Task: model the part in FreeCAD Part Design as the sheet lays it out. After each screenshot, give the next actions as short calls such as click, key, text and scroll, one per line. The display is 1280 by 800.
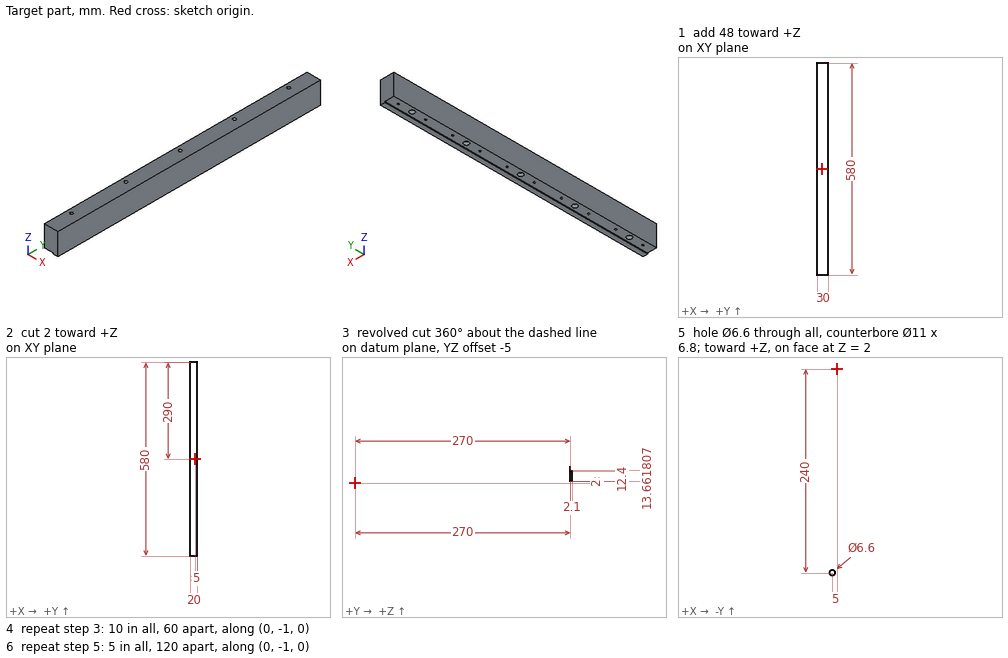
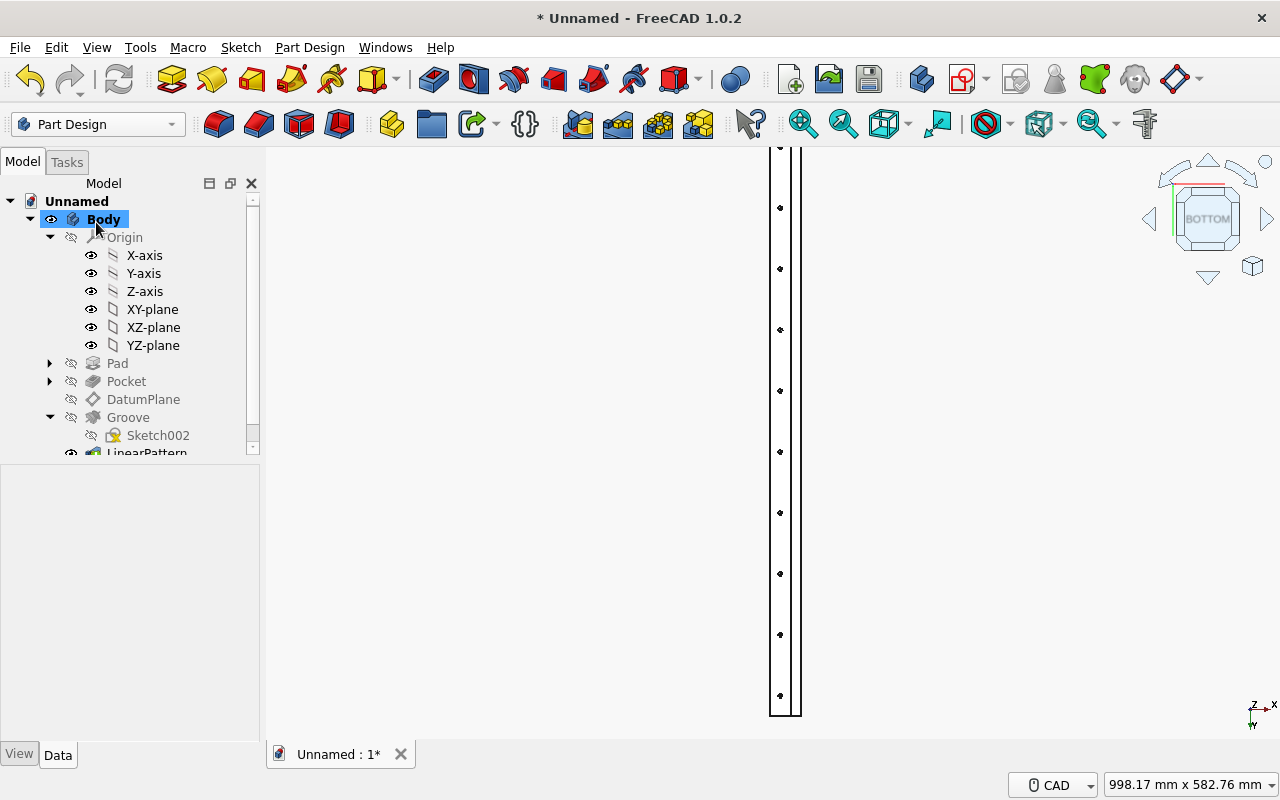
click(804, 124)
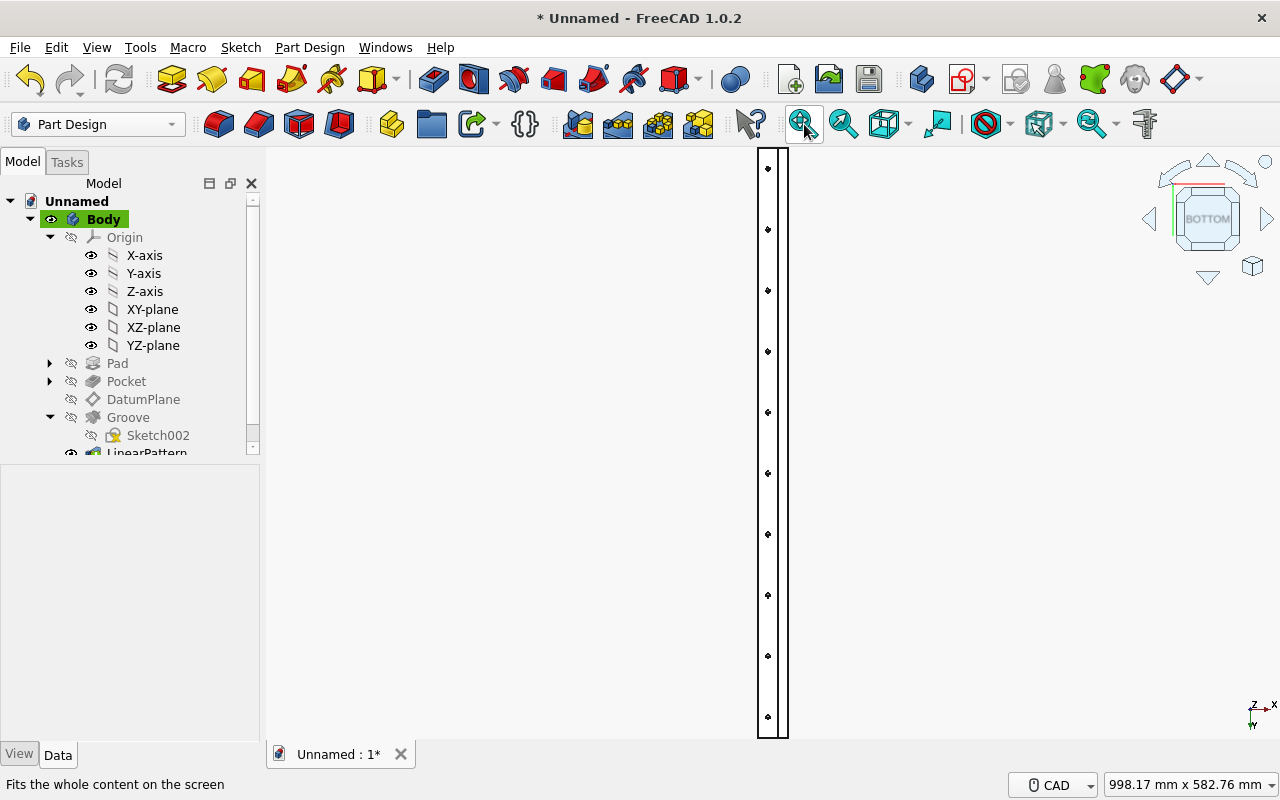
click(768, 695)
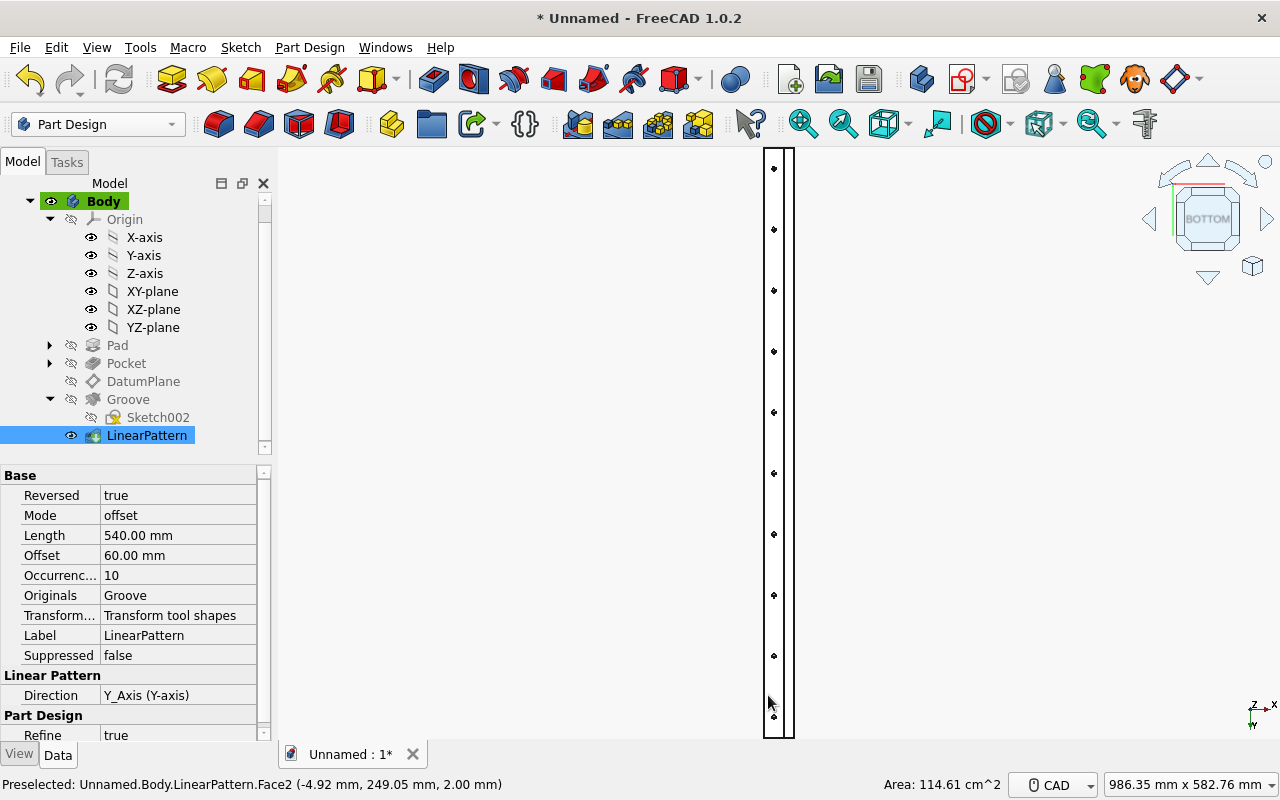
click(962, 80)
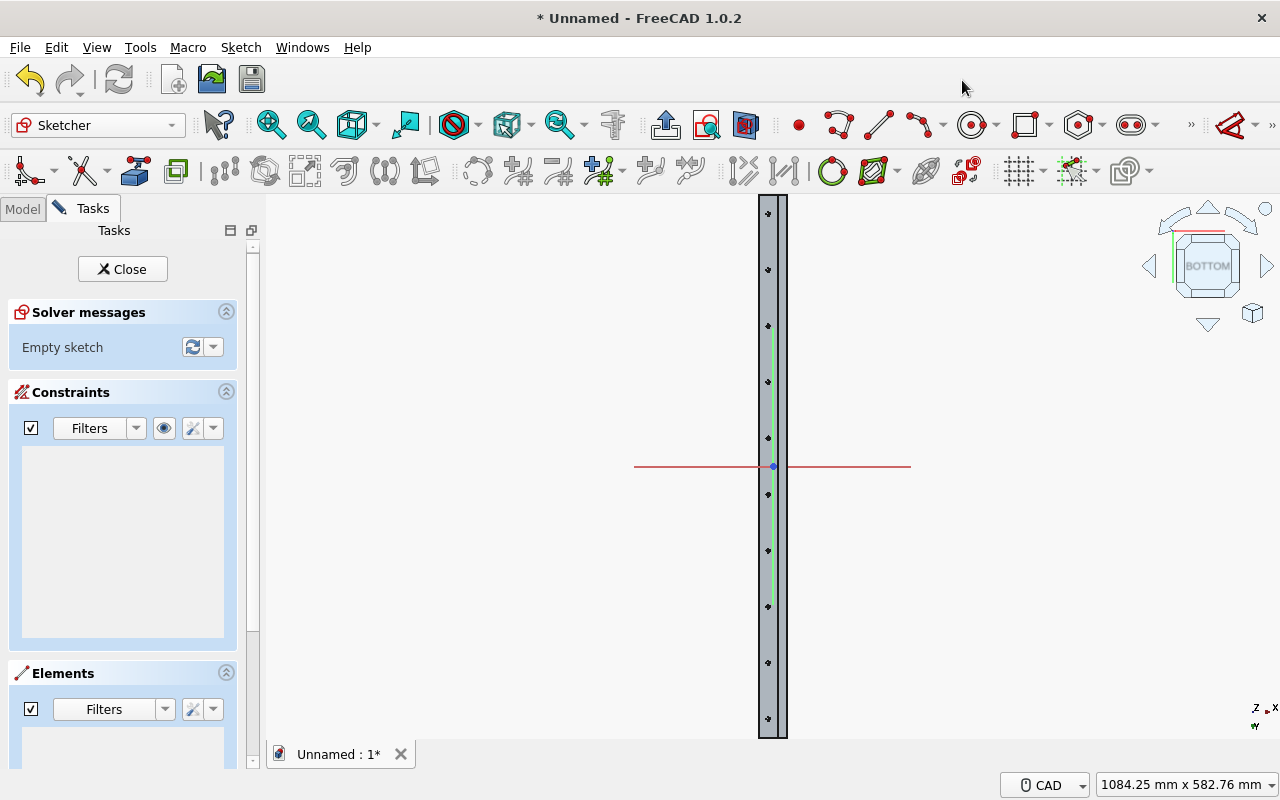
scroll(772, 703, up, 15)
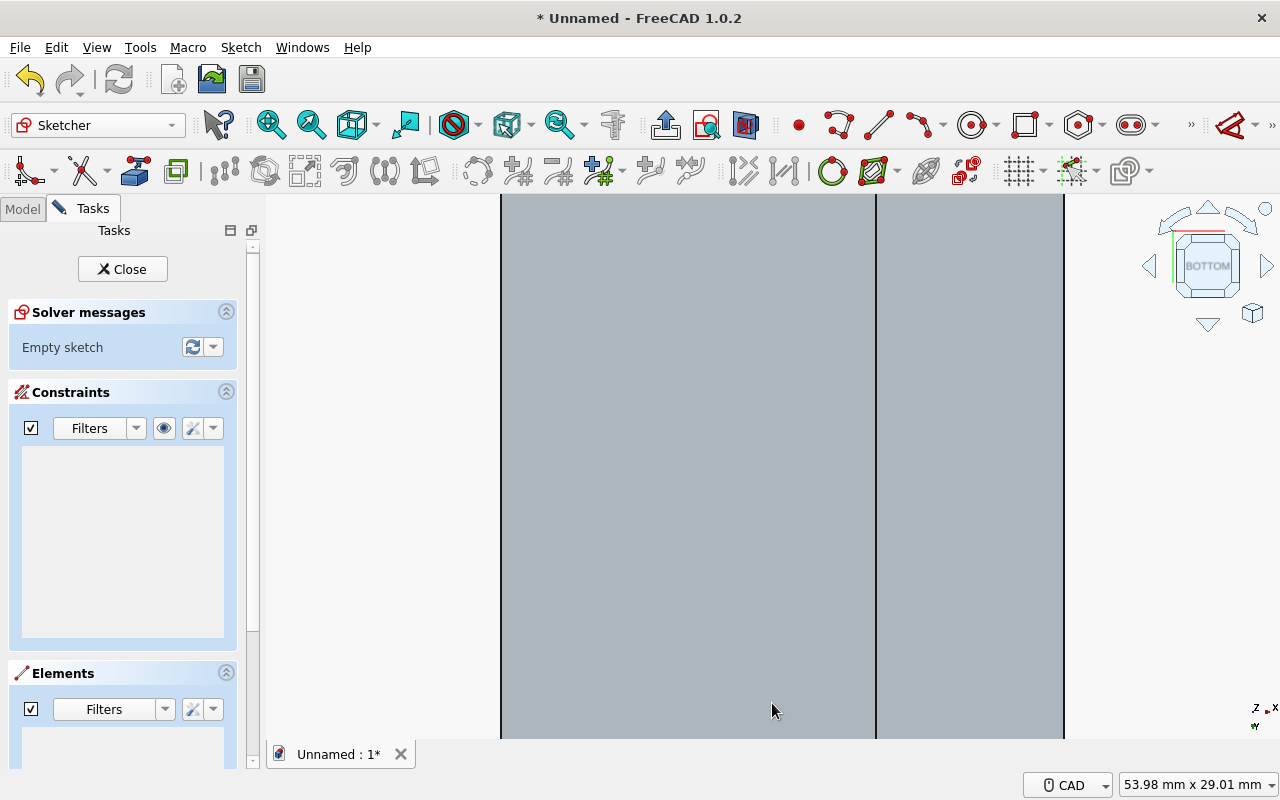
scroll(679, 430, up, 5)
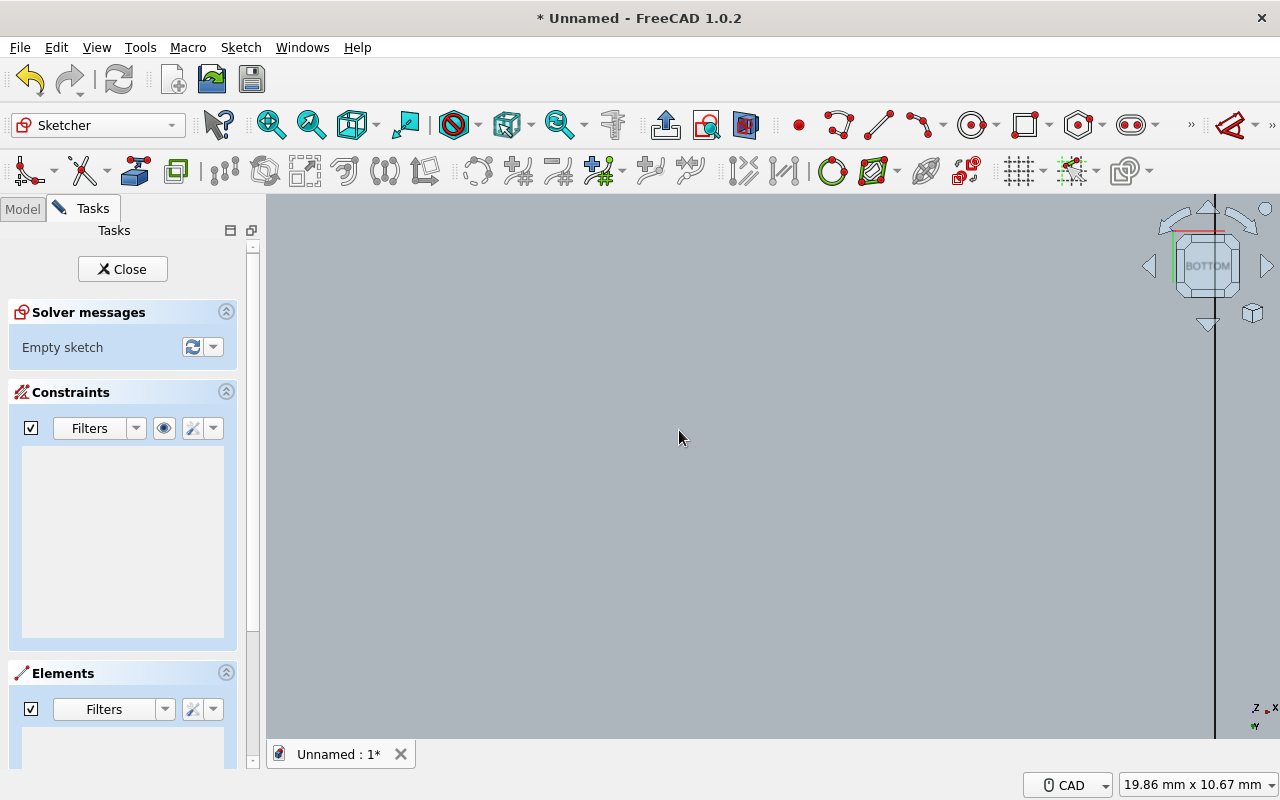
key(g)
key(c)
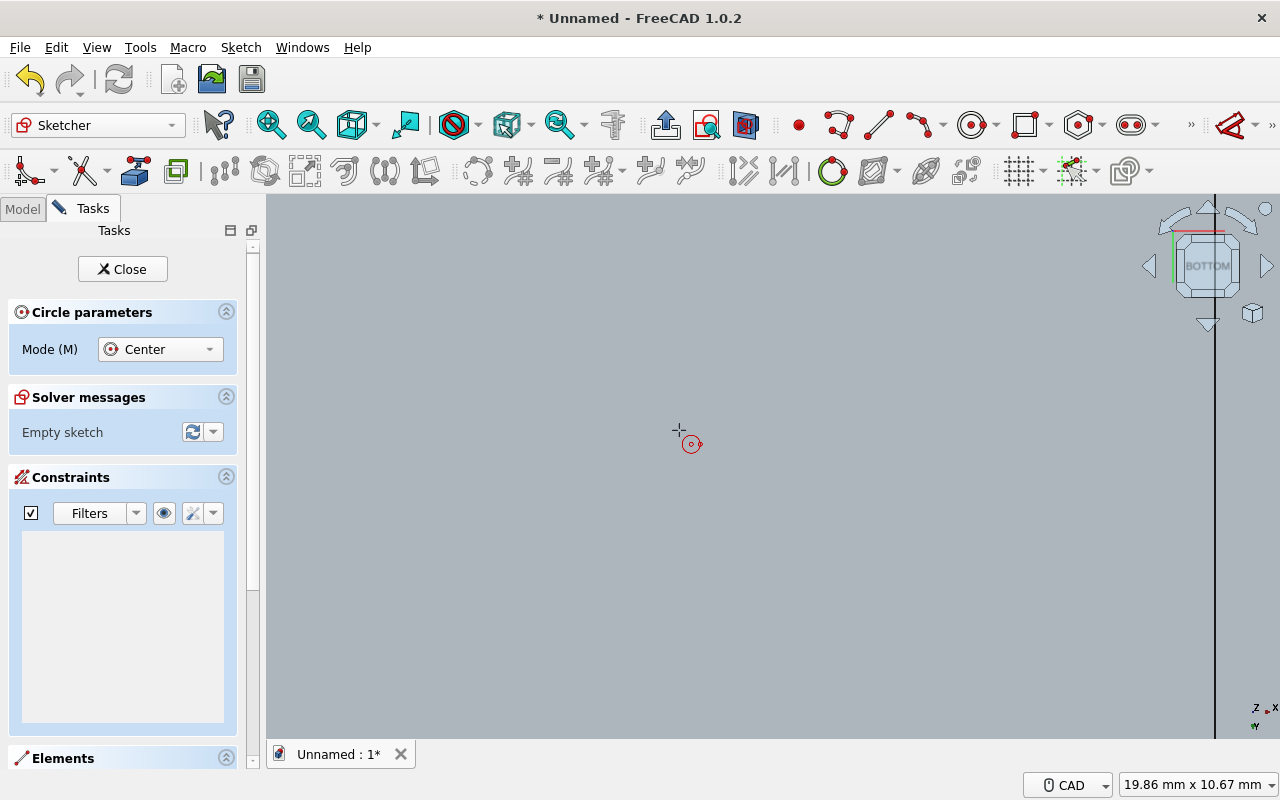
click(704, 465)
click(824, 346)
key(Escape)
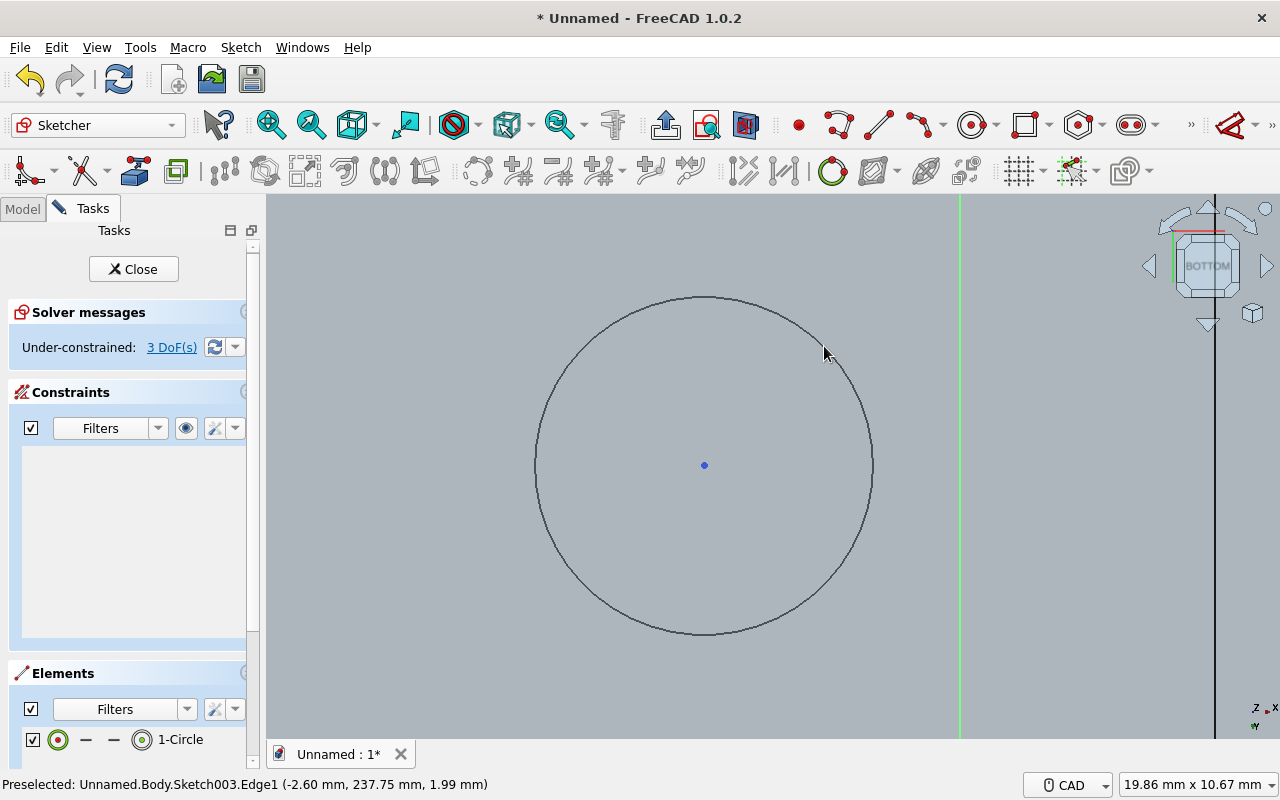
key(d)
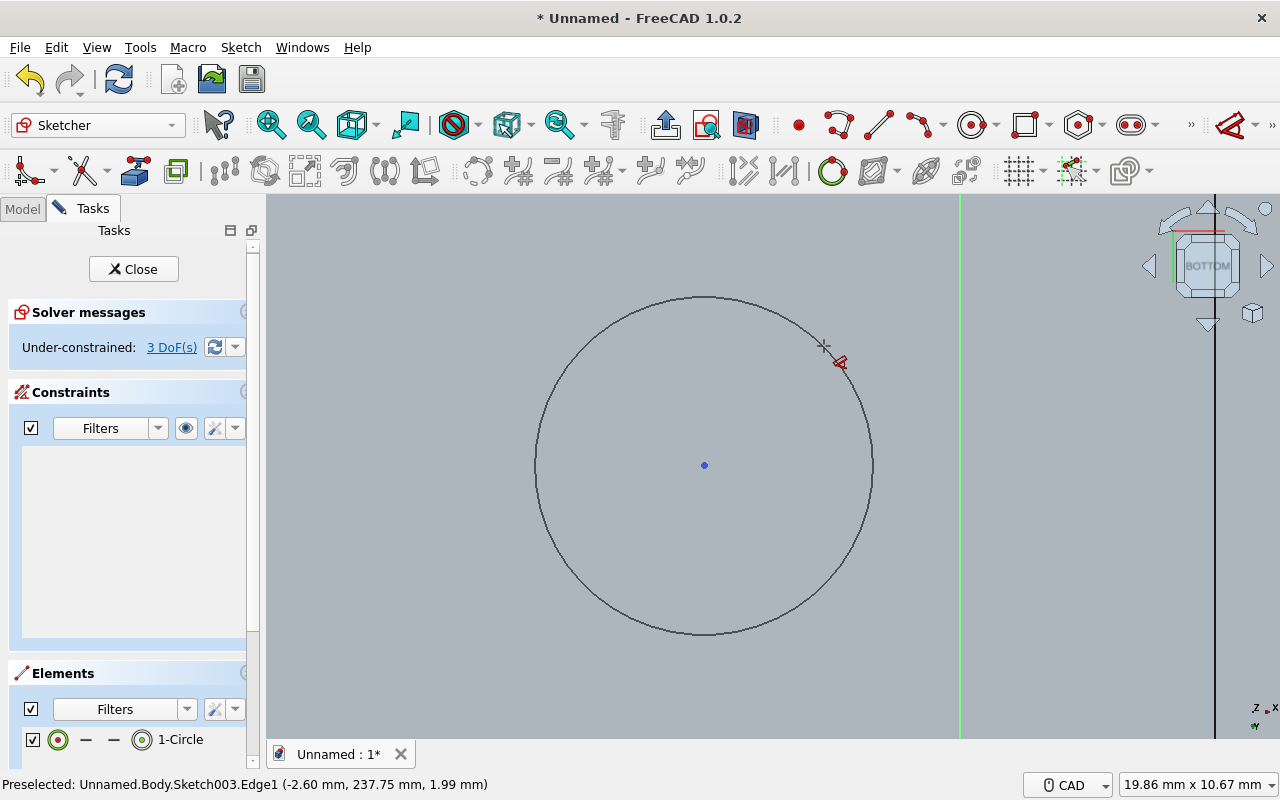
click(823, 346)
click(846, 323)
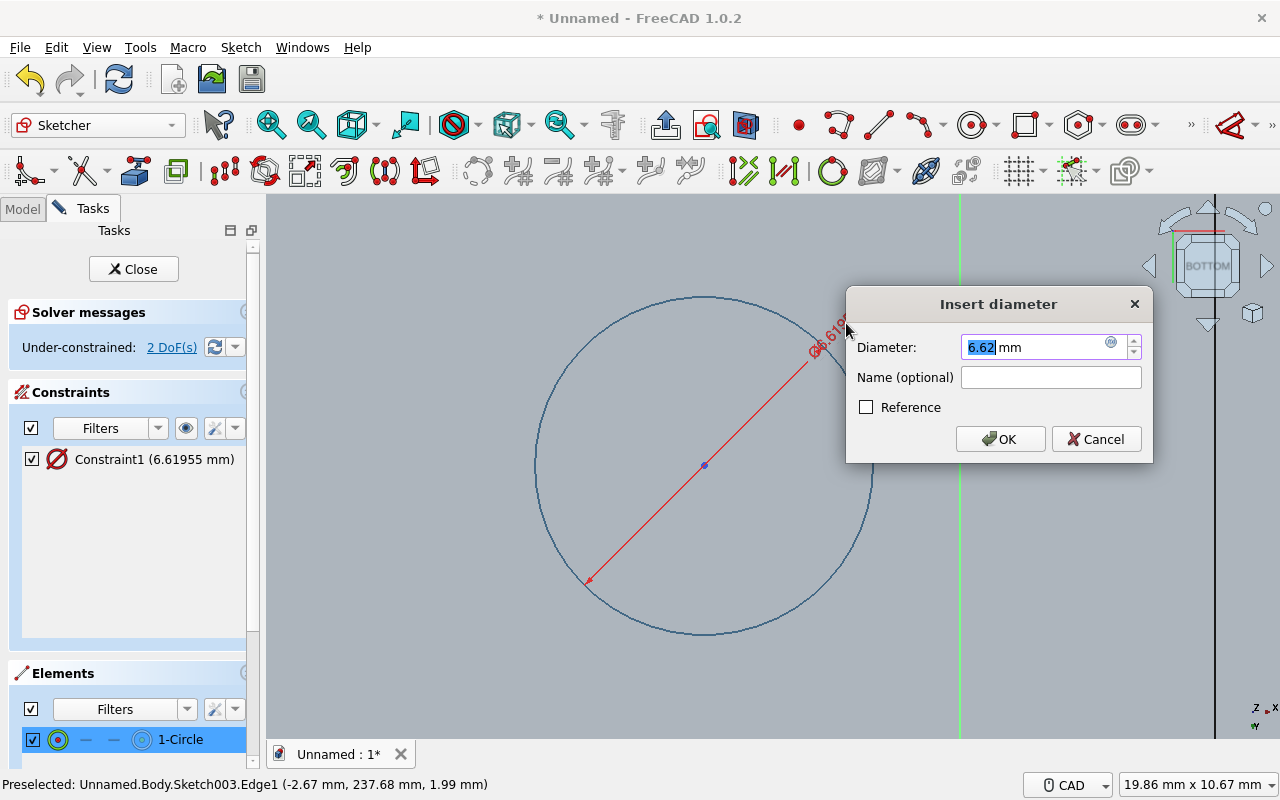
text(6.6)
key(Return)